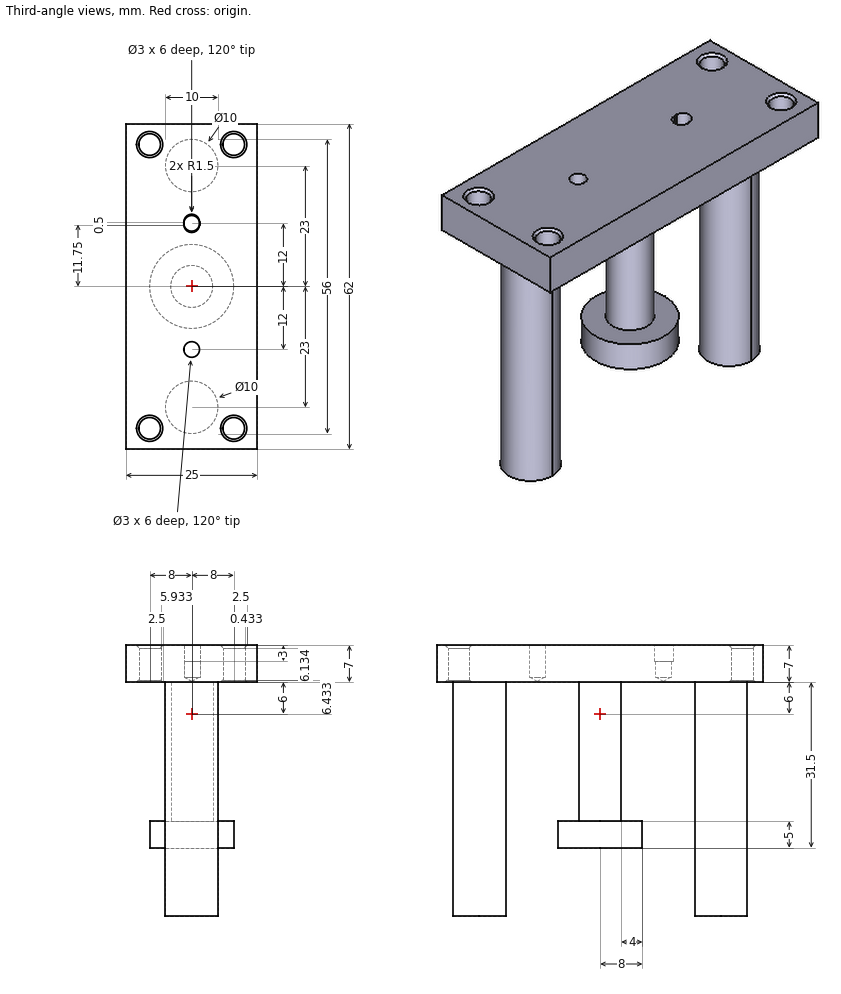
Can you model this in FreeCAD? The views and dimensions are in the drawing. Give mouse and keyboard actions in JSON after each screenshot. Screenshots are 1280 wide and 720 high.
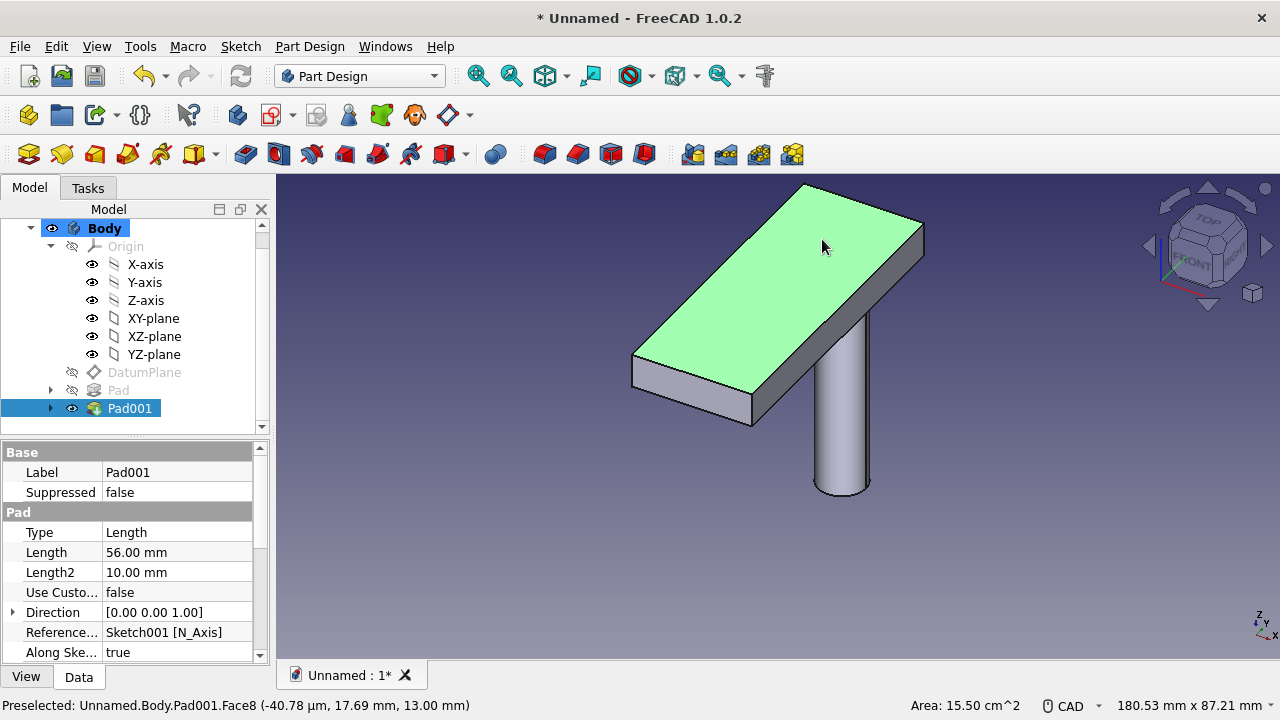
{"action": "left_click", "coordinate": [270, 116]}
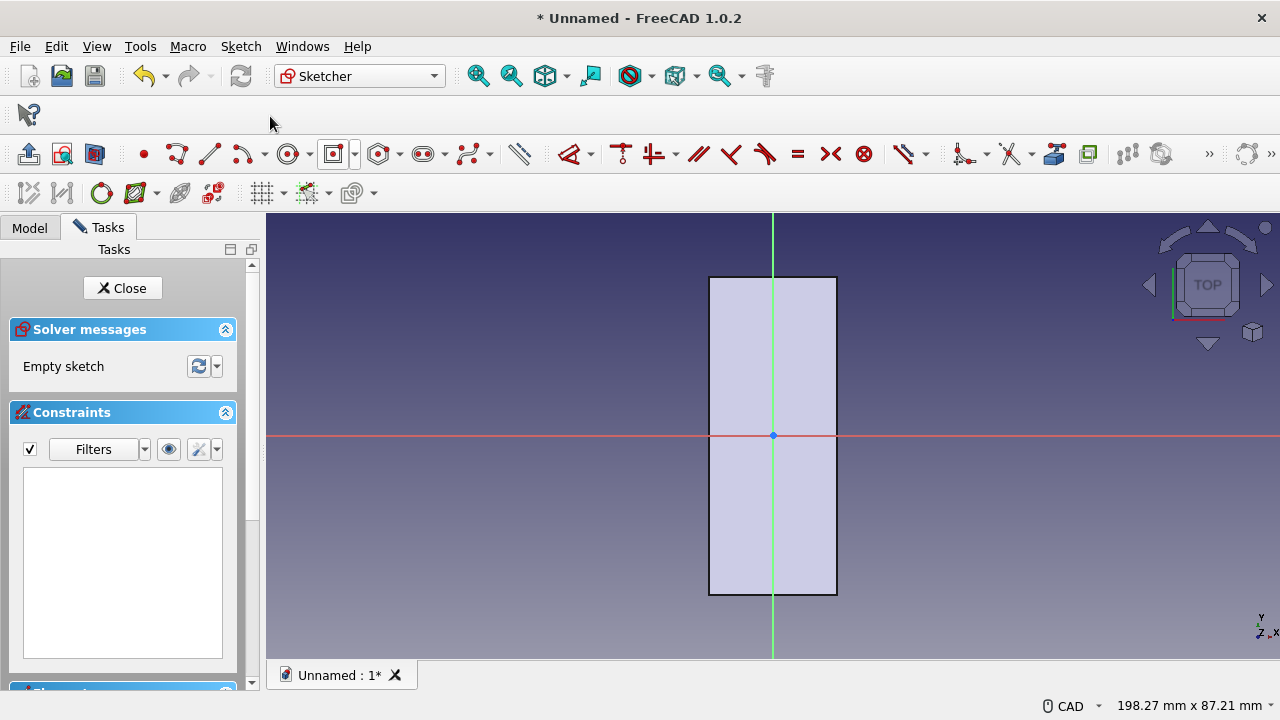
{"action": "scroll", "coordinate": [790, 583], "scroll_direction": "up", "scroll_amount": 8}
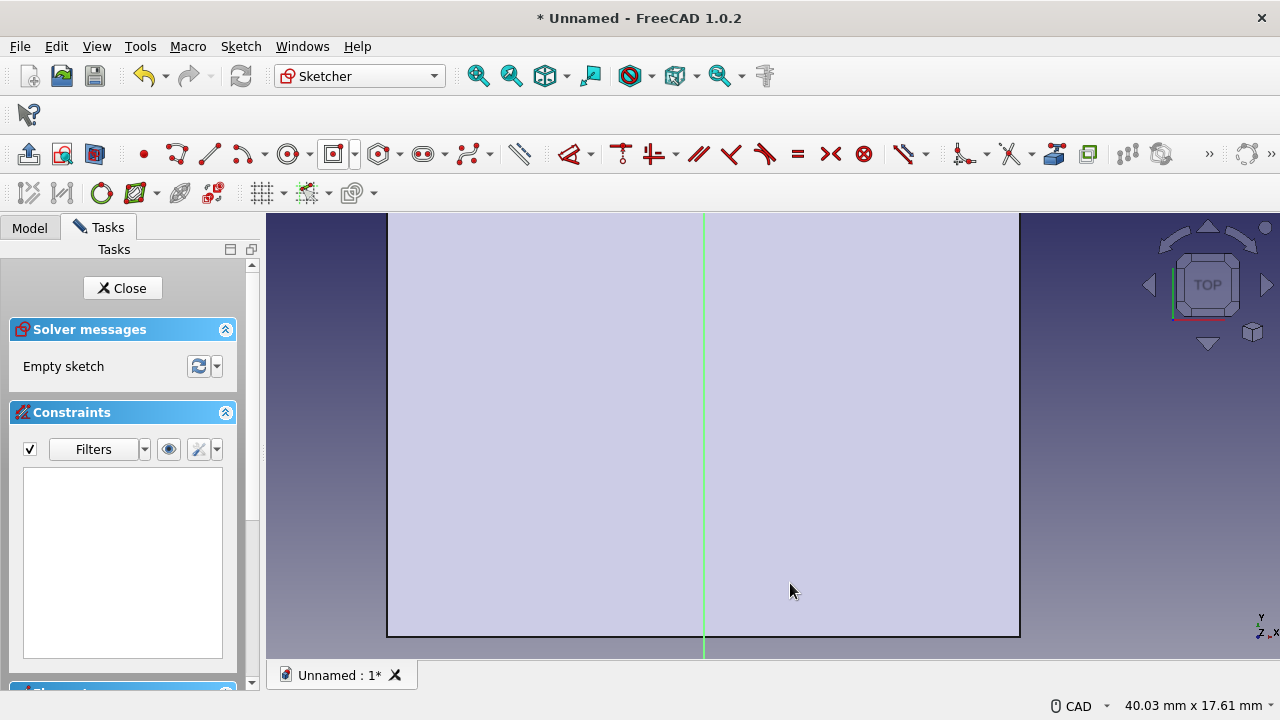
{"action": "left_click", "coordinate": [288, 154]}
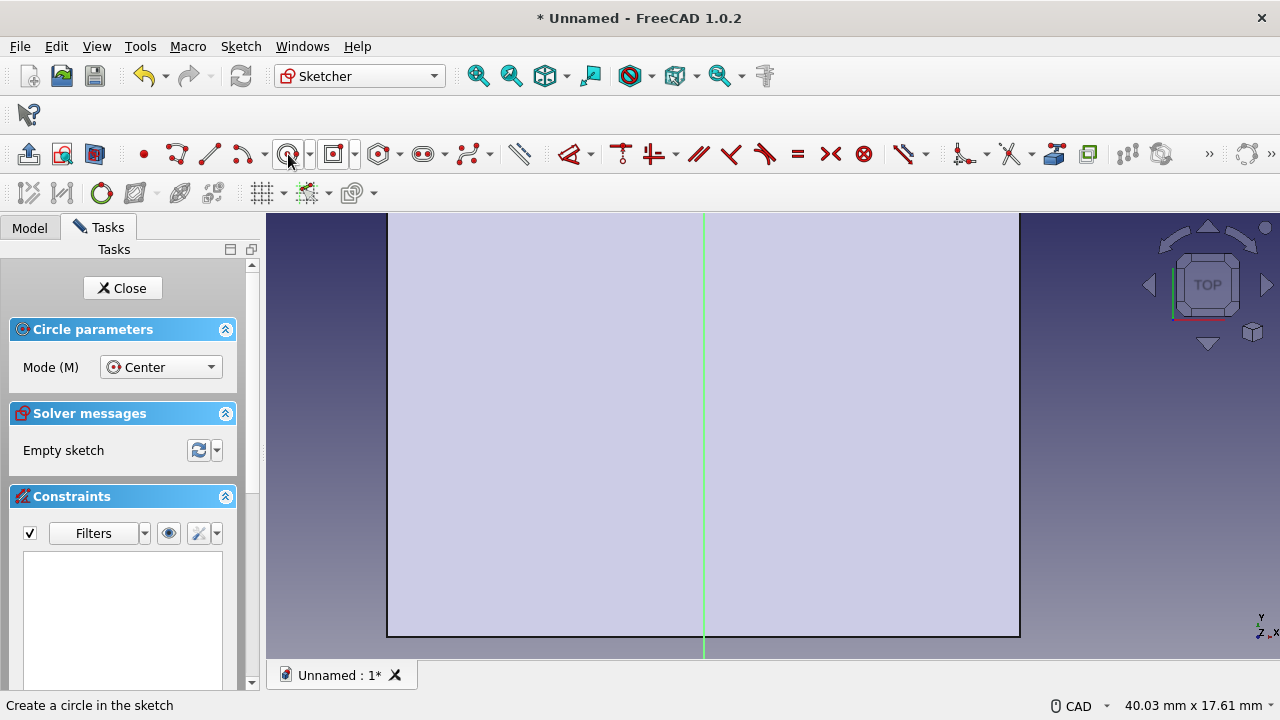
{"action": "left_click", "coordinate": [704, 434]}
{"action": "left_click", "coordinate": [793, 345]}
{"action": "key", "text": "Escape"}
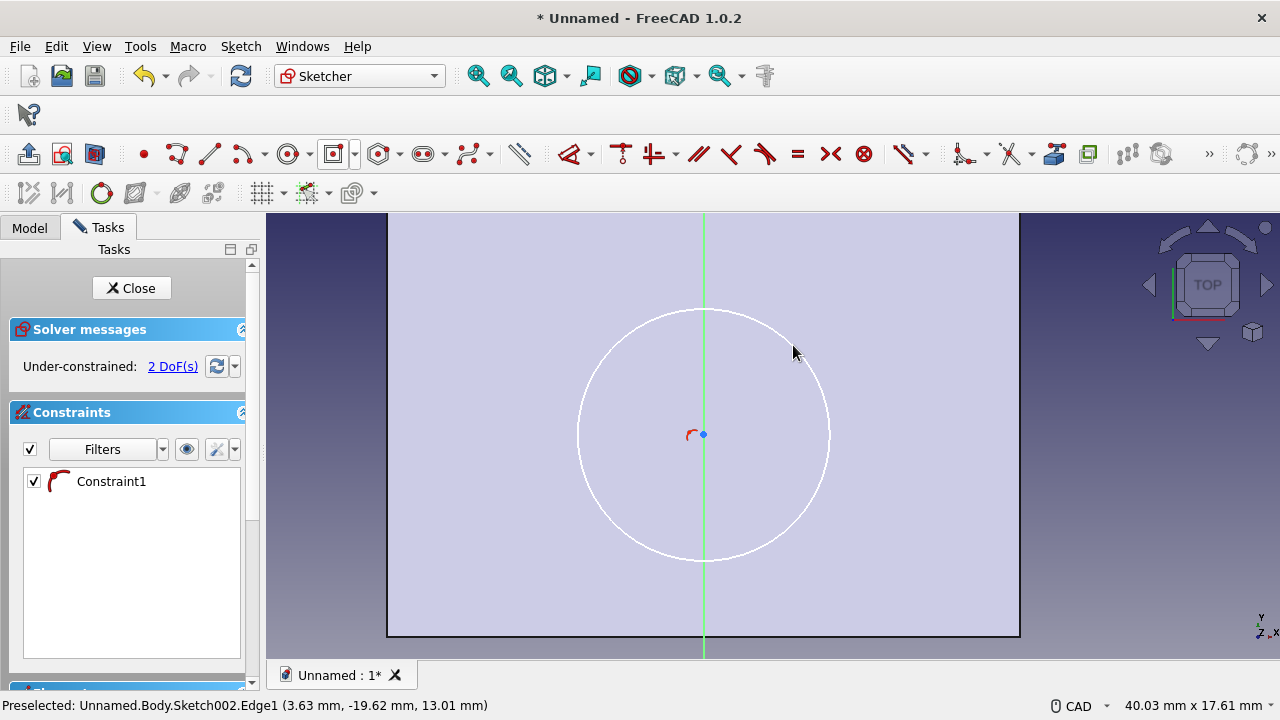
{"action": "left_click", "coordinate": [568, 154]}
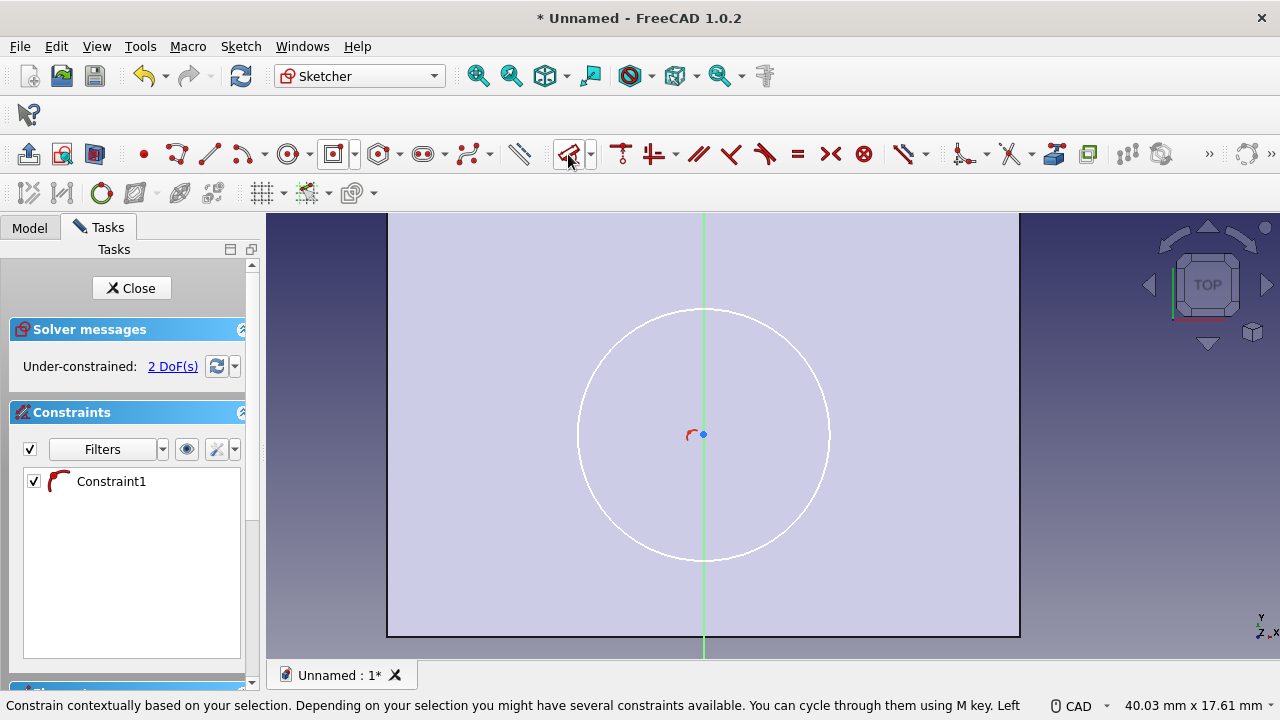
{"action": "left_click", "coordinate": [793, 346]}
{"action": "left_click", "coordinate": [816, 323]}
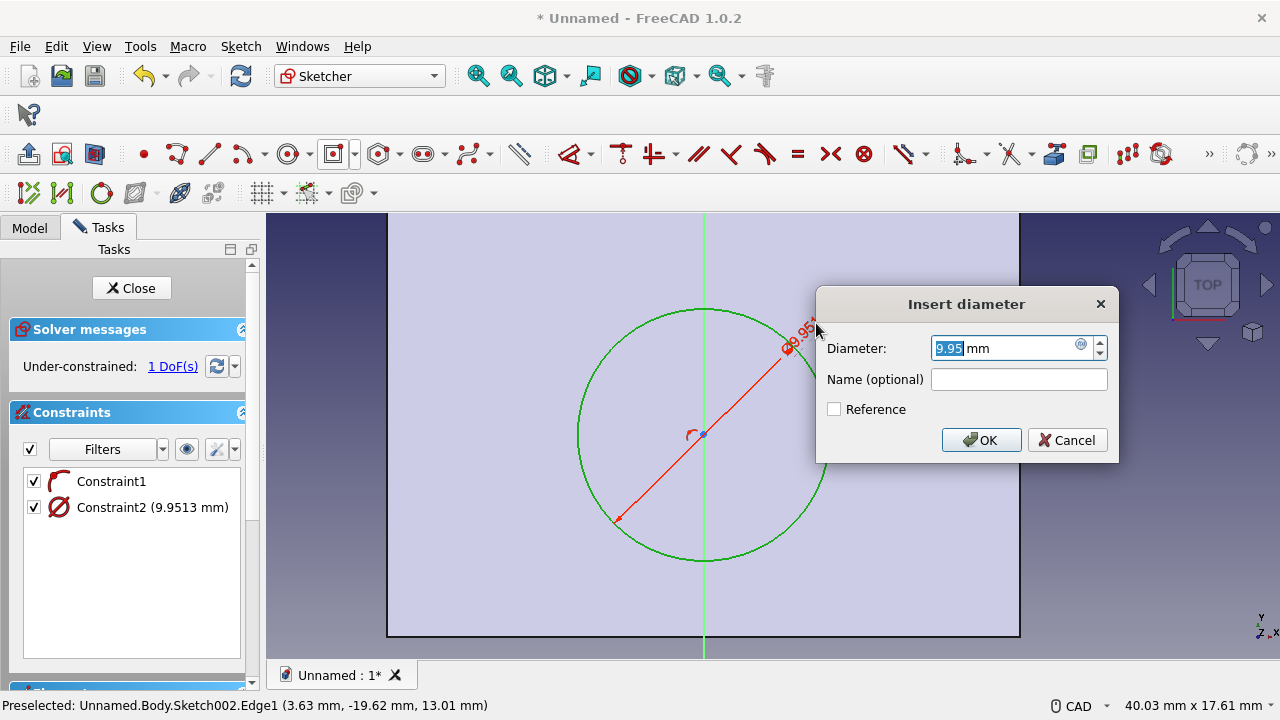
{"action": "type", "text": "10"}
{"action": "key", "text": "Return"}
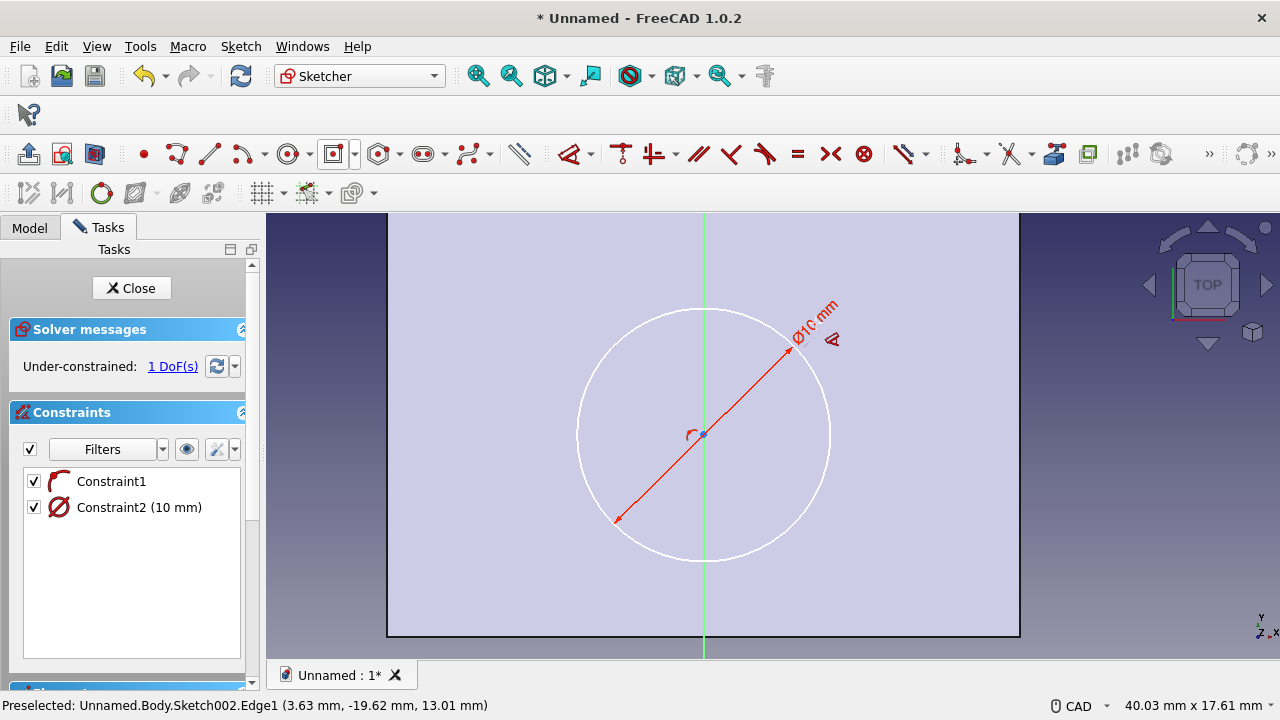
{"action": "left_click", "coordinate": [704, 435]}
{"action": "left_click", "coordinate": [738, 338]}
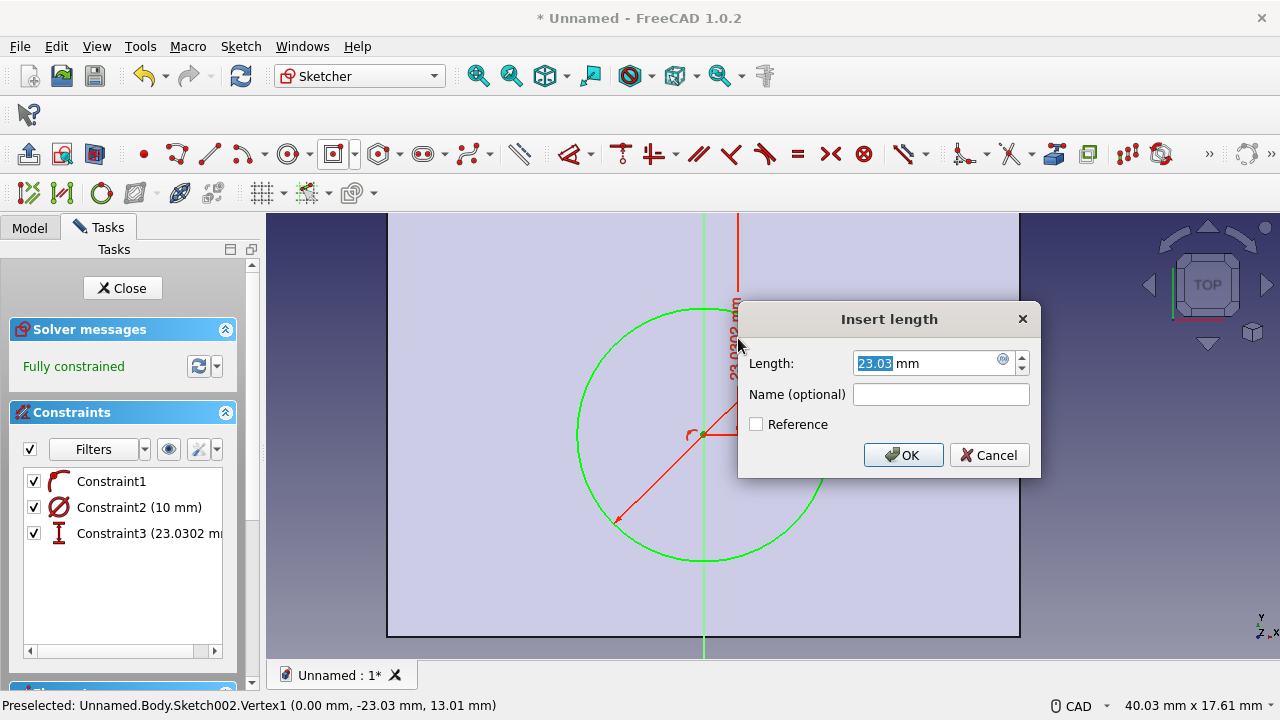
{"action": "type", "text": "23"}
{"action": "key", "text": "Return"}
{"action": "key", "text": "Escape"}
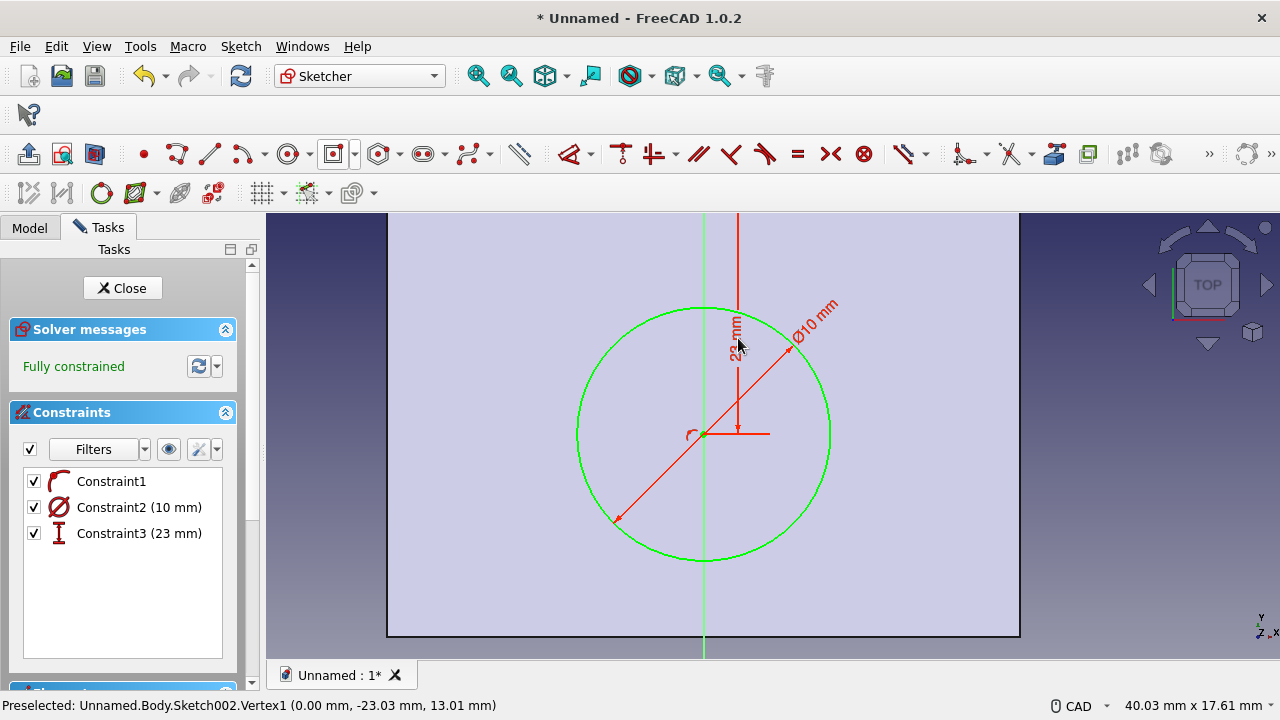
{"action": "left_click", "coordinate": [123, 288]}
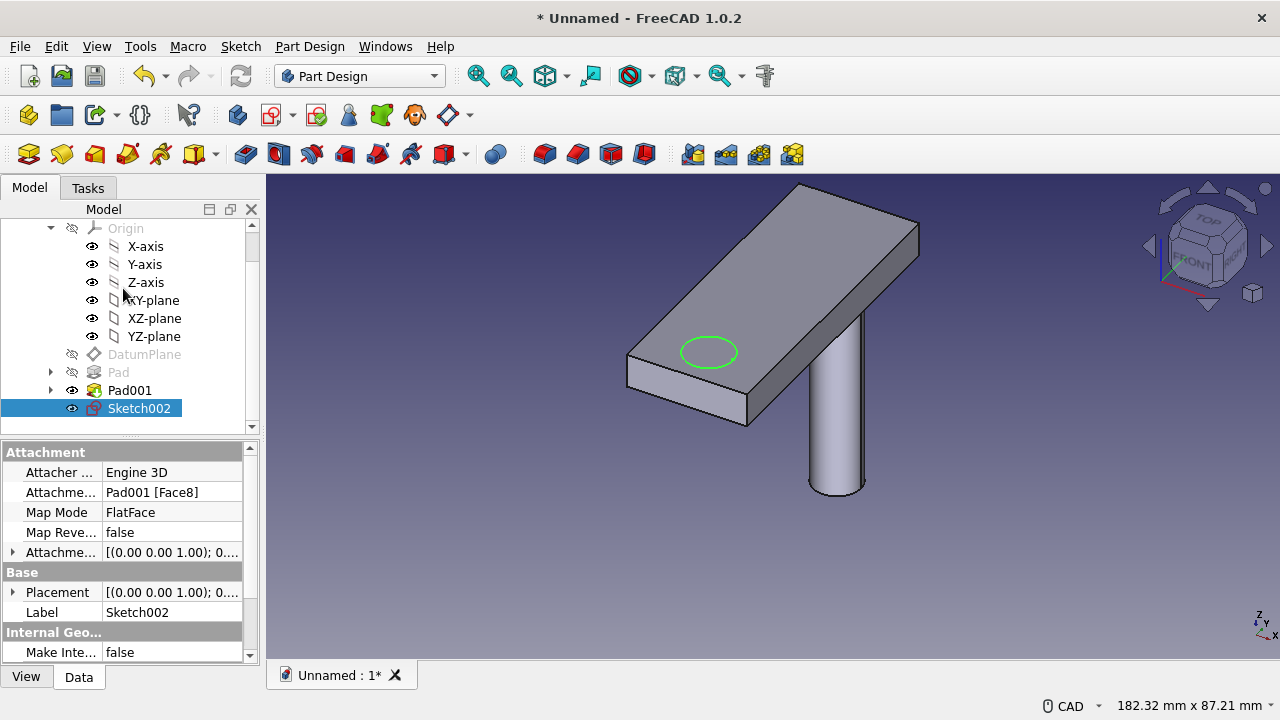
{"action": "left_click", "coordinate": [29, 154]}